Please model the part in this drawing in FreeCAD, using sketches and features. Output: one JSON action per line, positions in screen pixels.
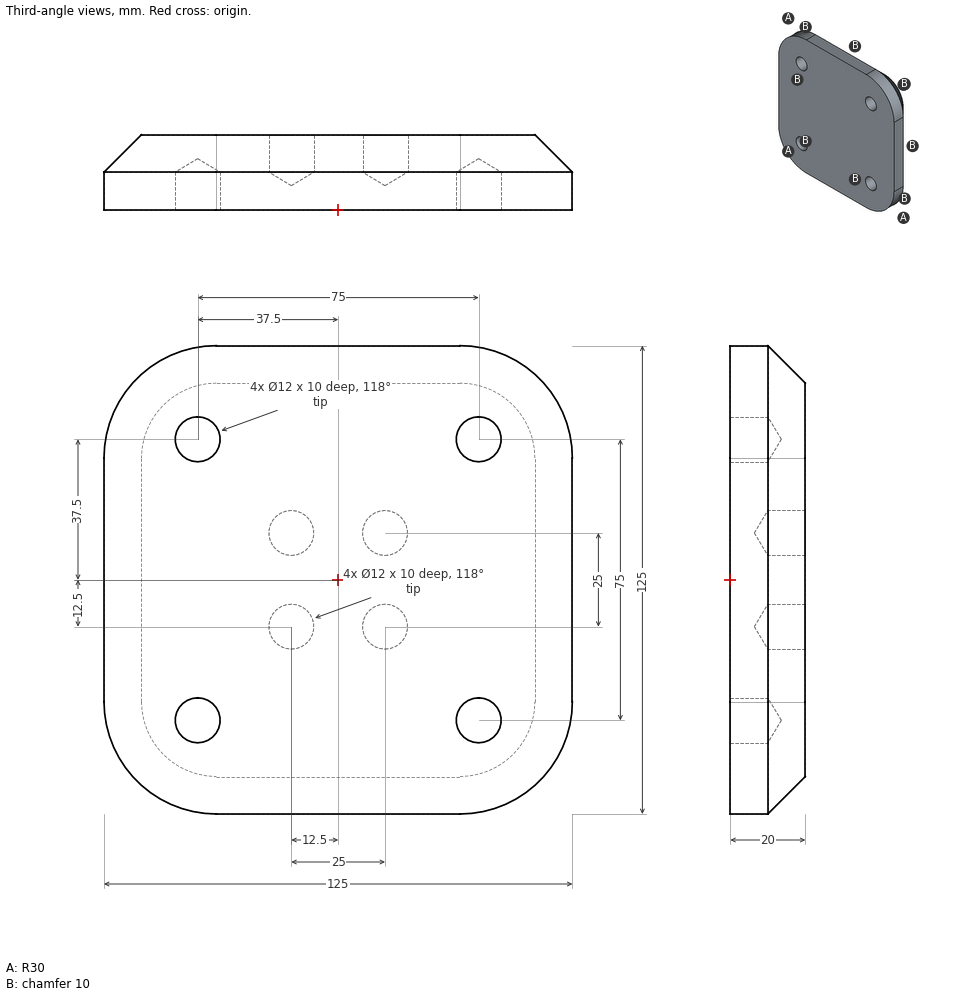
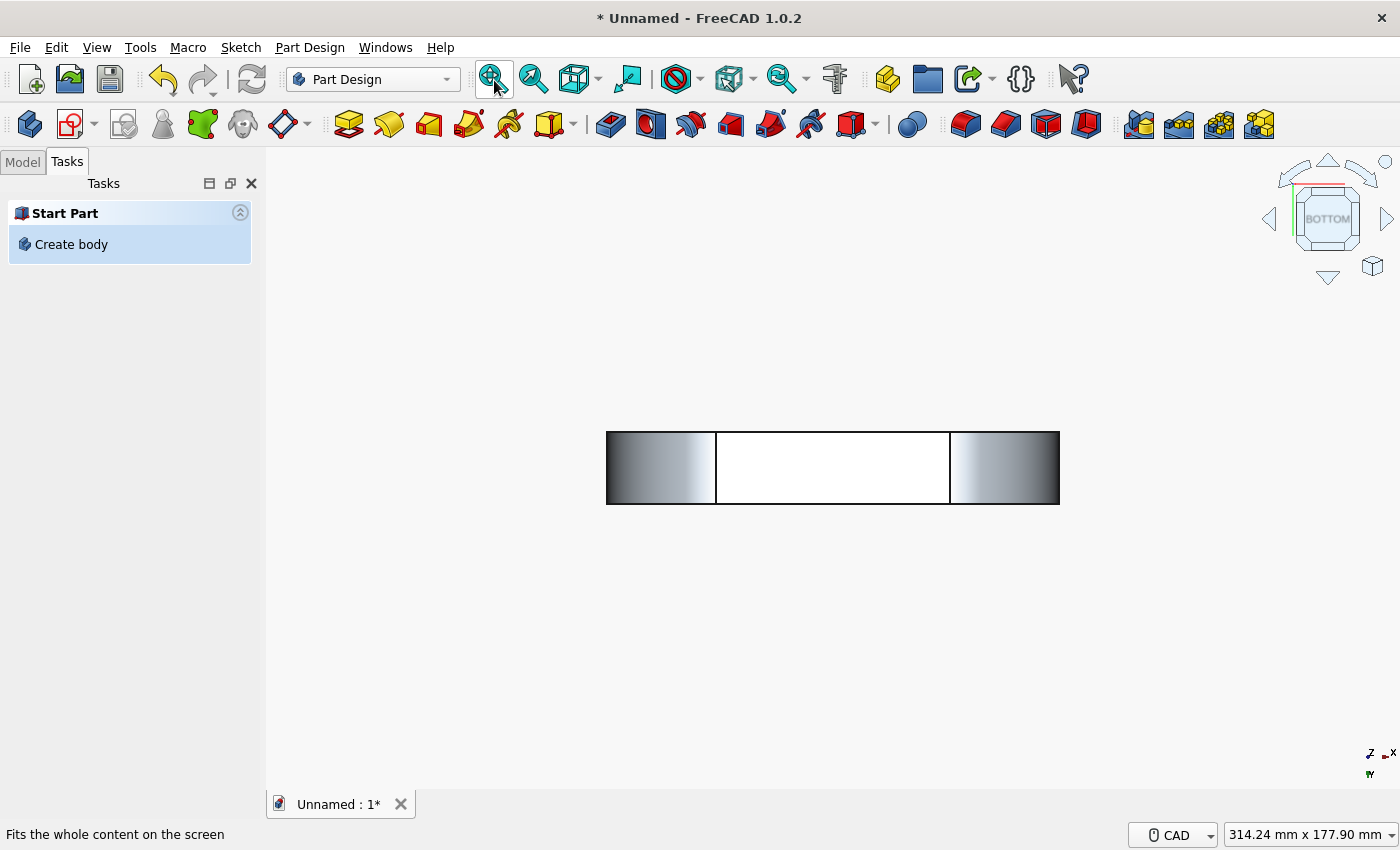
{"action": "key", "text": "v f"}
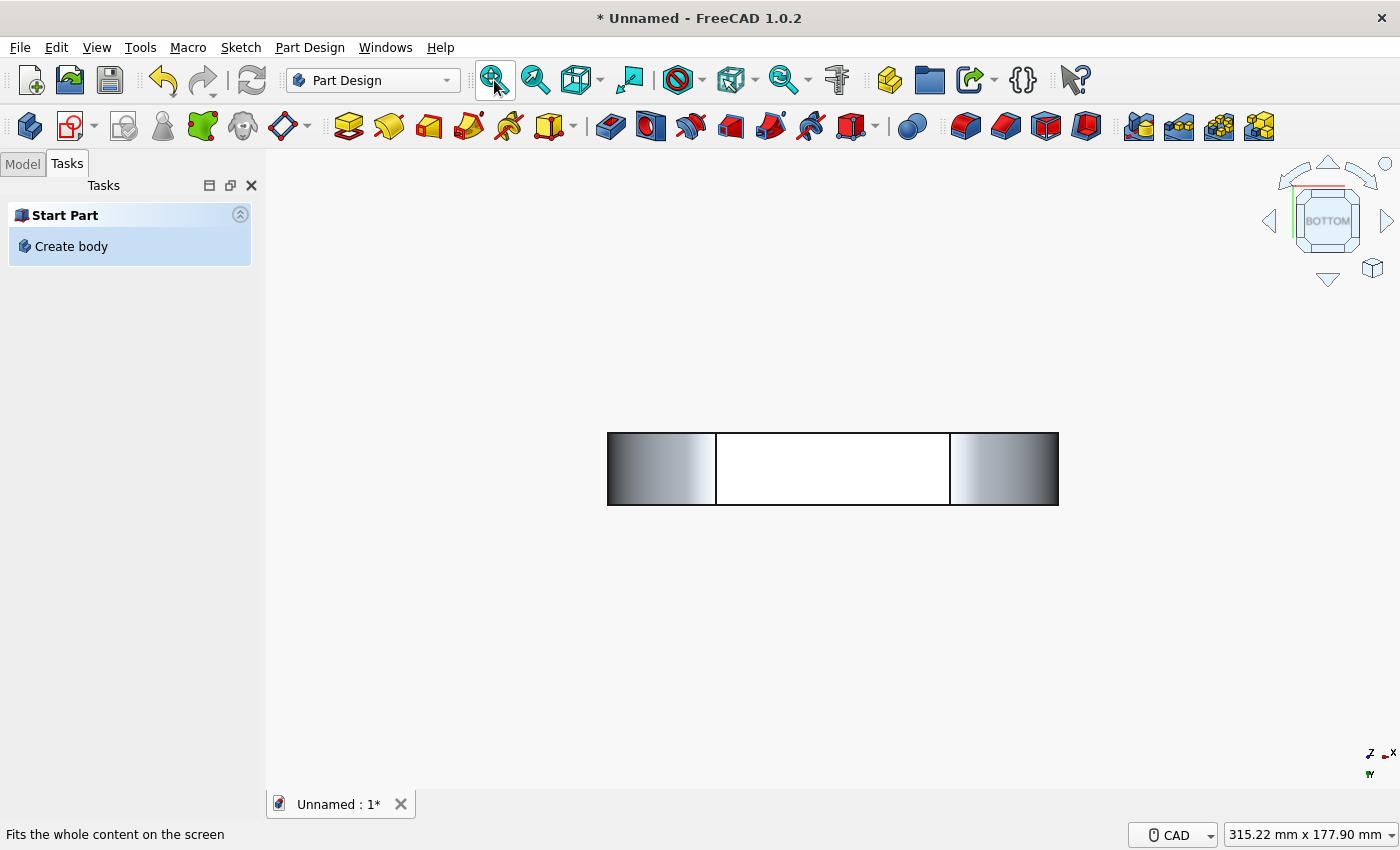
{"action": "key", "text": "4"}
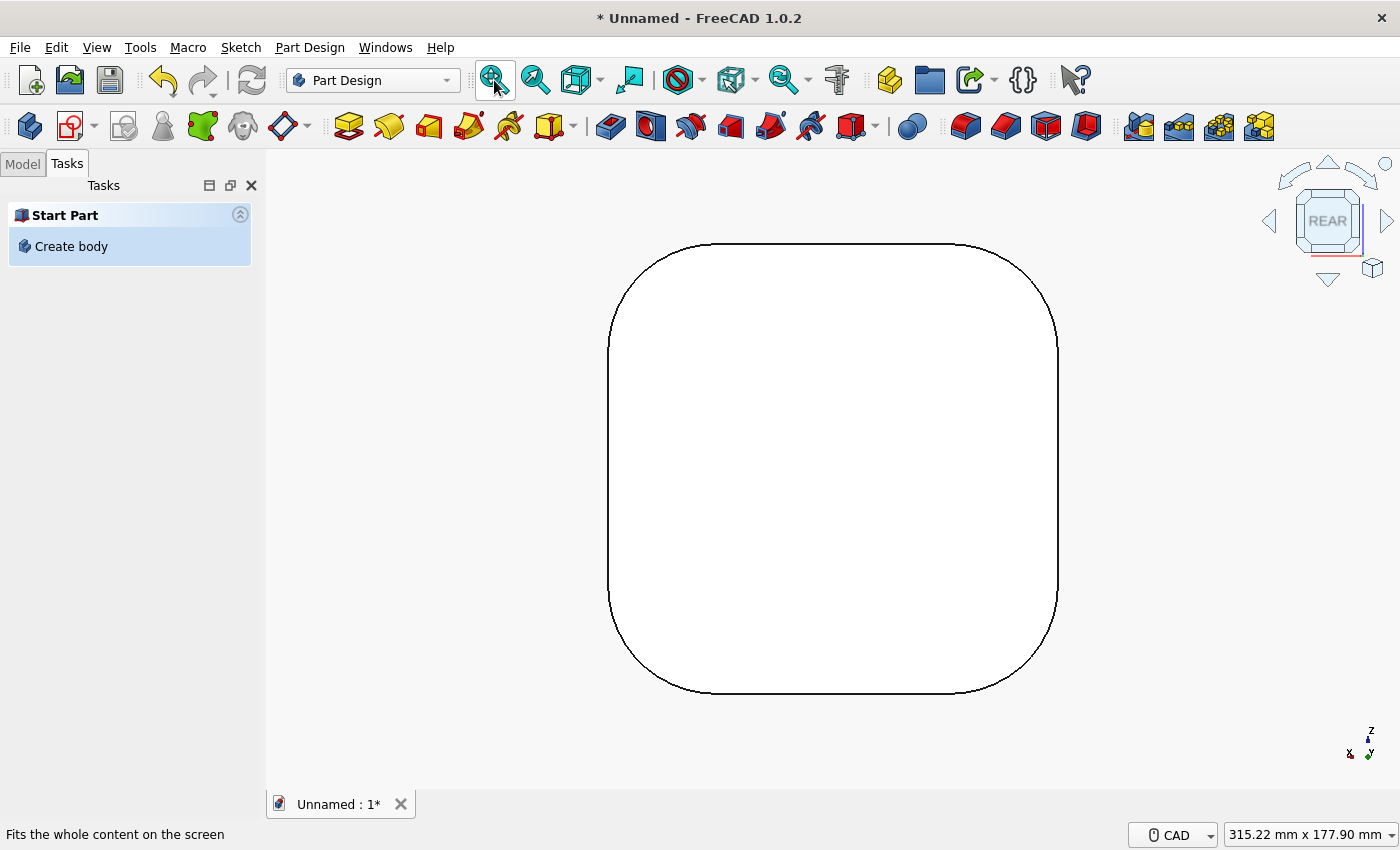
{"action": "left_click", "coordinate": [833, 468]}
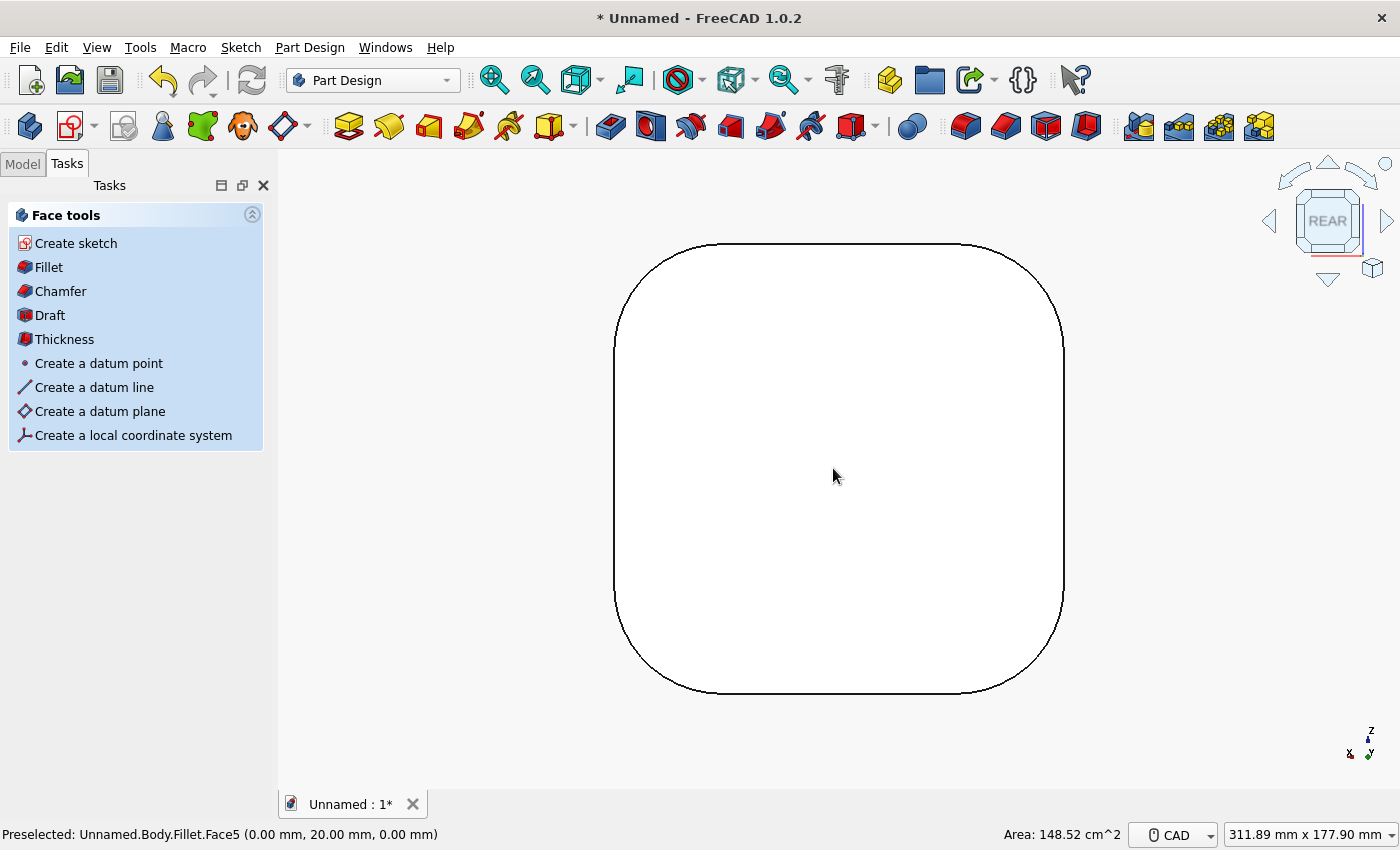
{"action": "left_click", "coordinate": [1006, 126]}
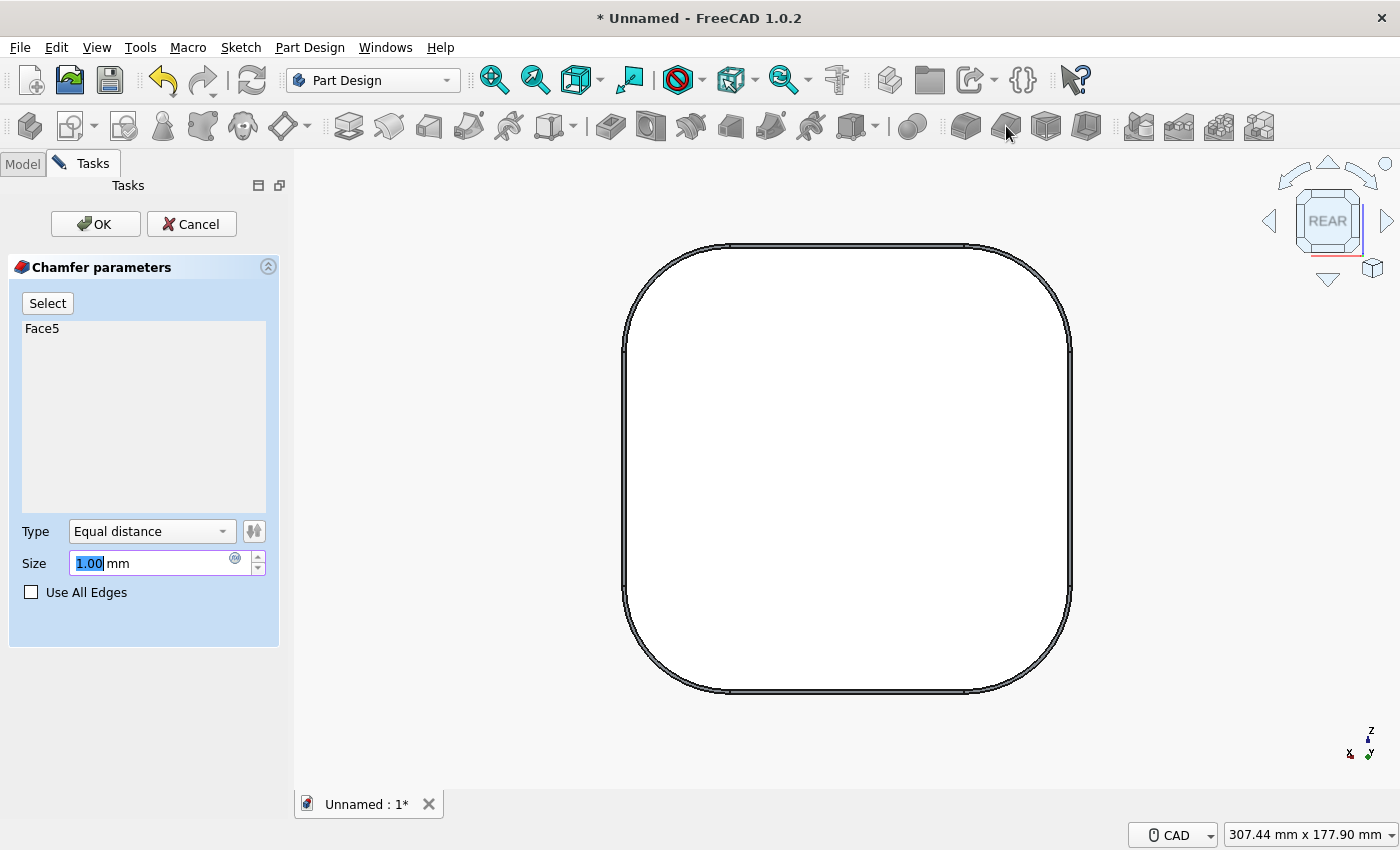
{"action": "type", "text": "10"}
{"action": "key", "text": "Tab"}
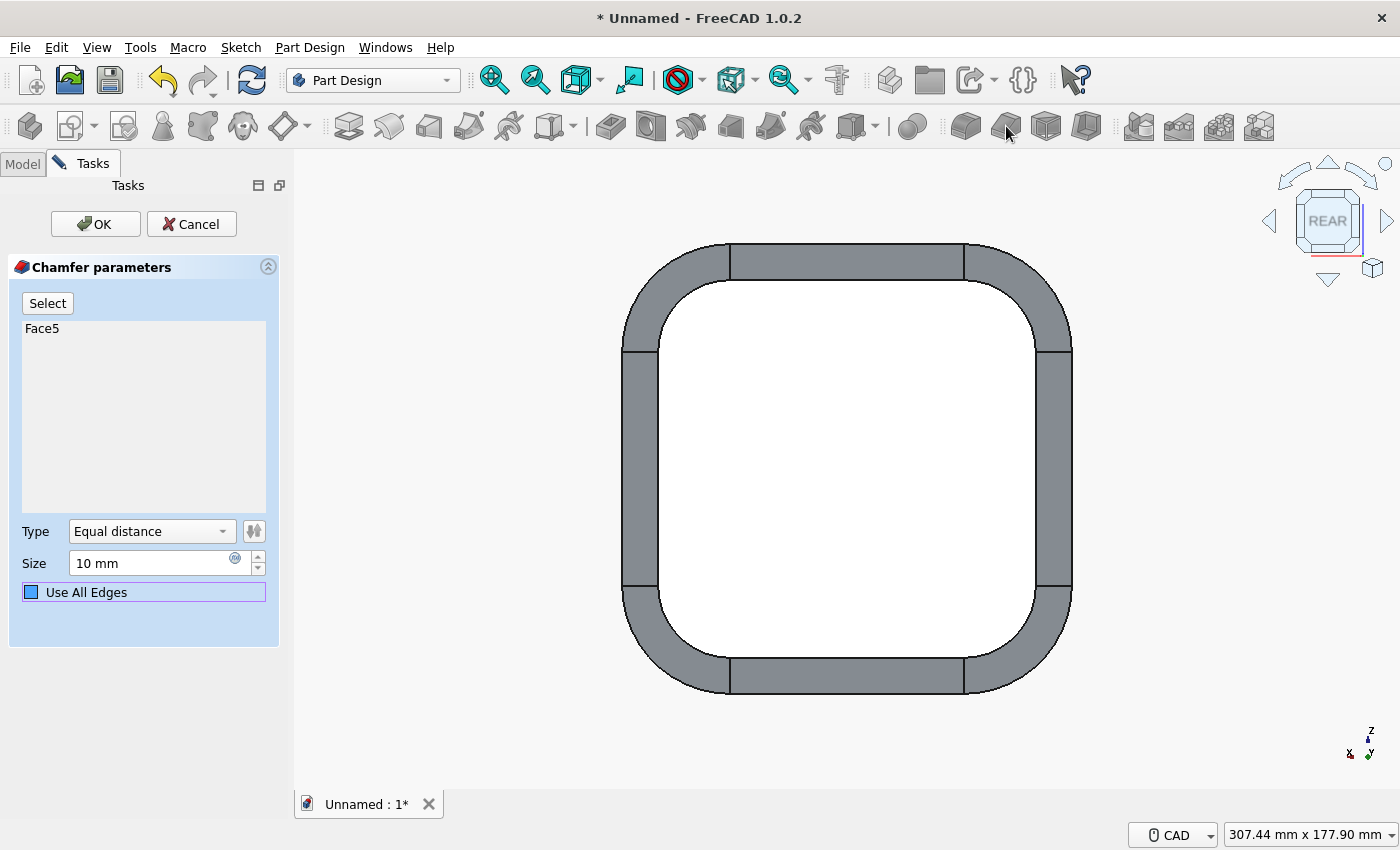
{"action": "left_click", "coordinate": [96, 224]}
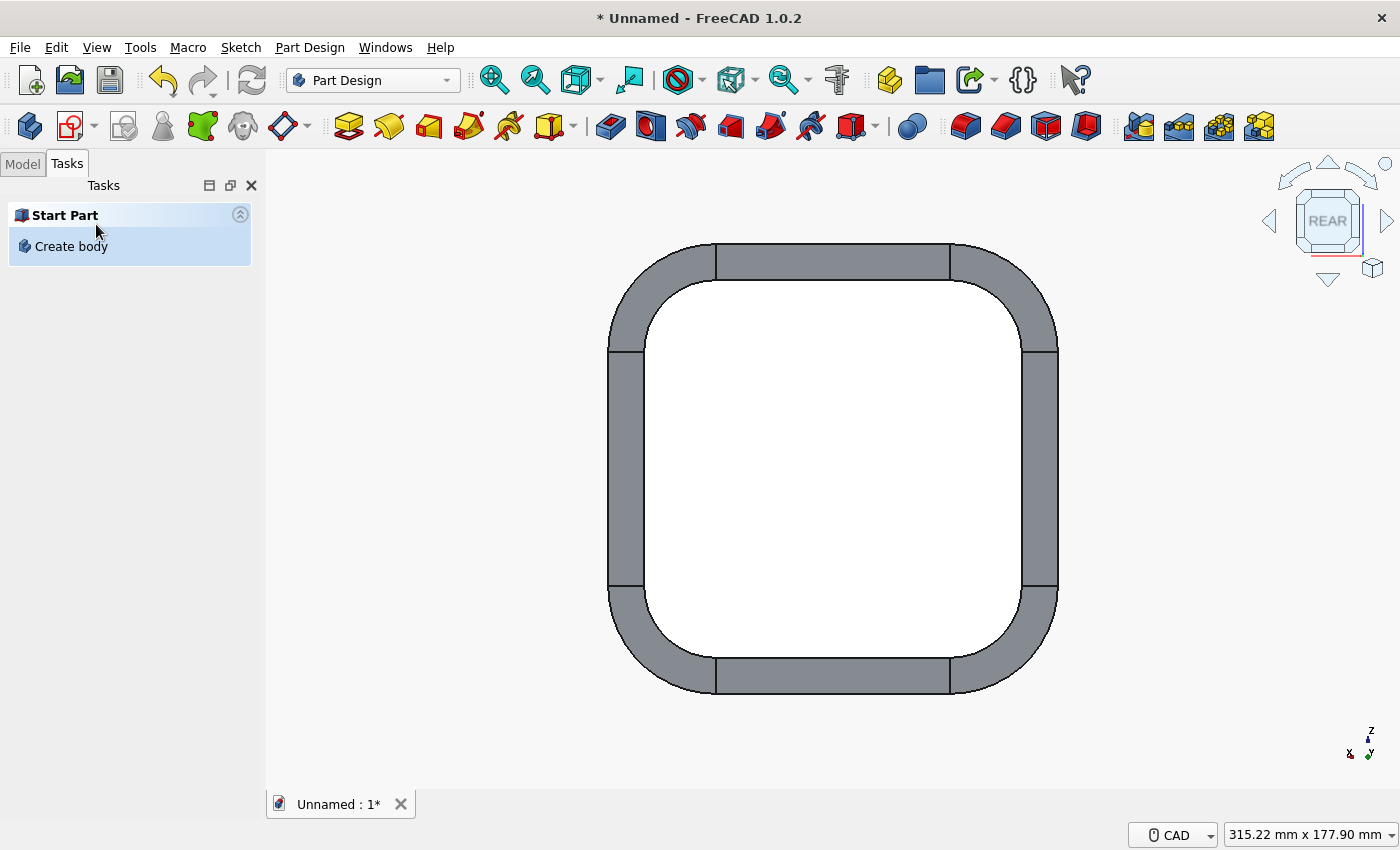
{"action": "left_click", "coordinate": [833, 468]}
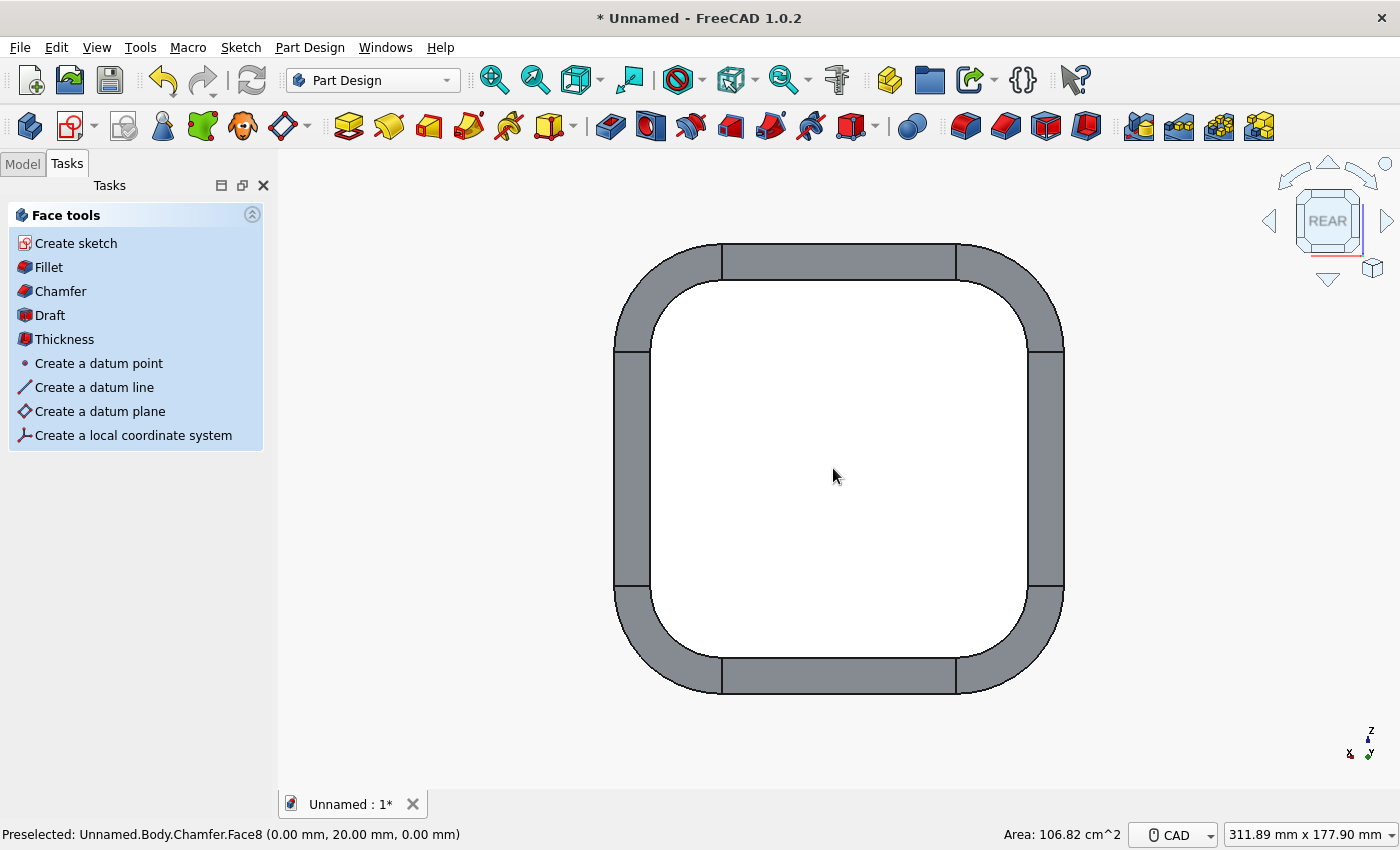
{"action": "left_click", "coordinate": [70, 126]}